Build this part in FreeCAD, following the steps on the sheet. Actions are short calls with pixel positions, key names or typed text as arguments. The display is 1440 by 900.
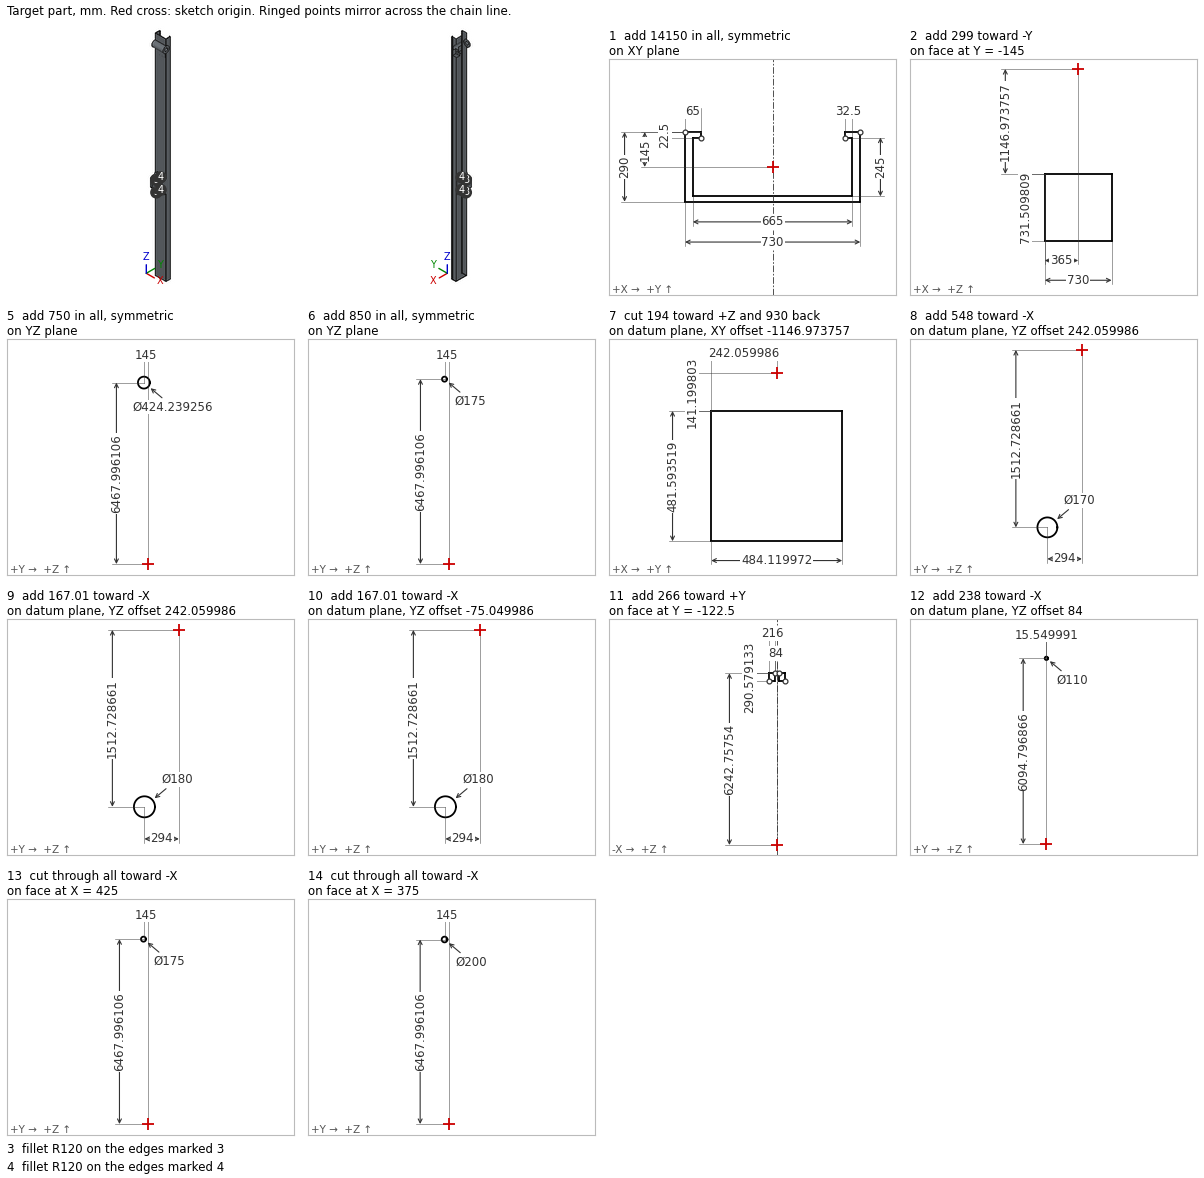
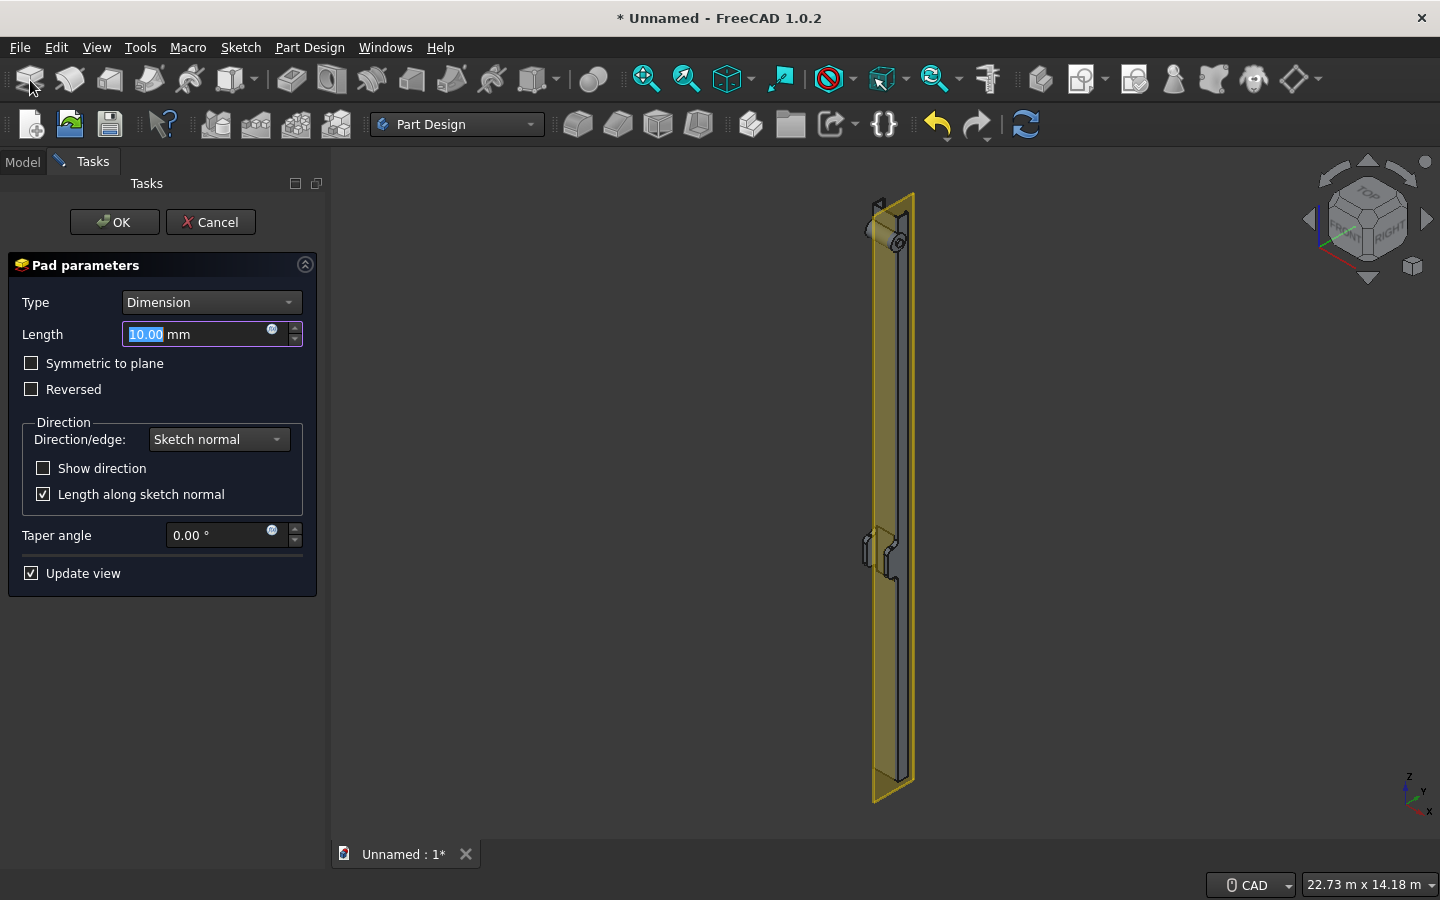
text(548)
key(Tab)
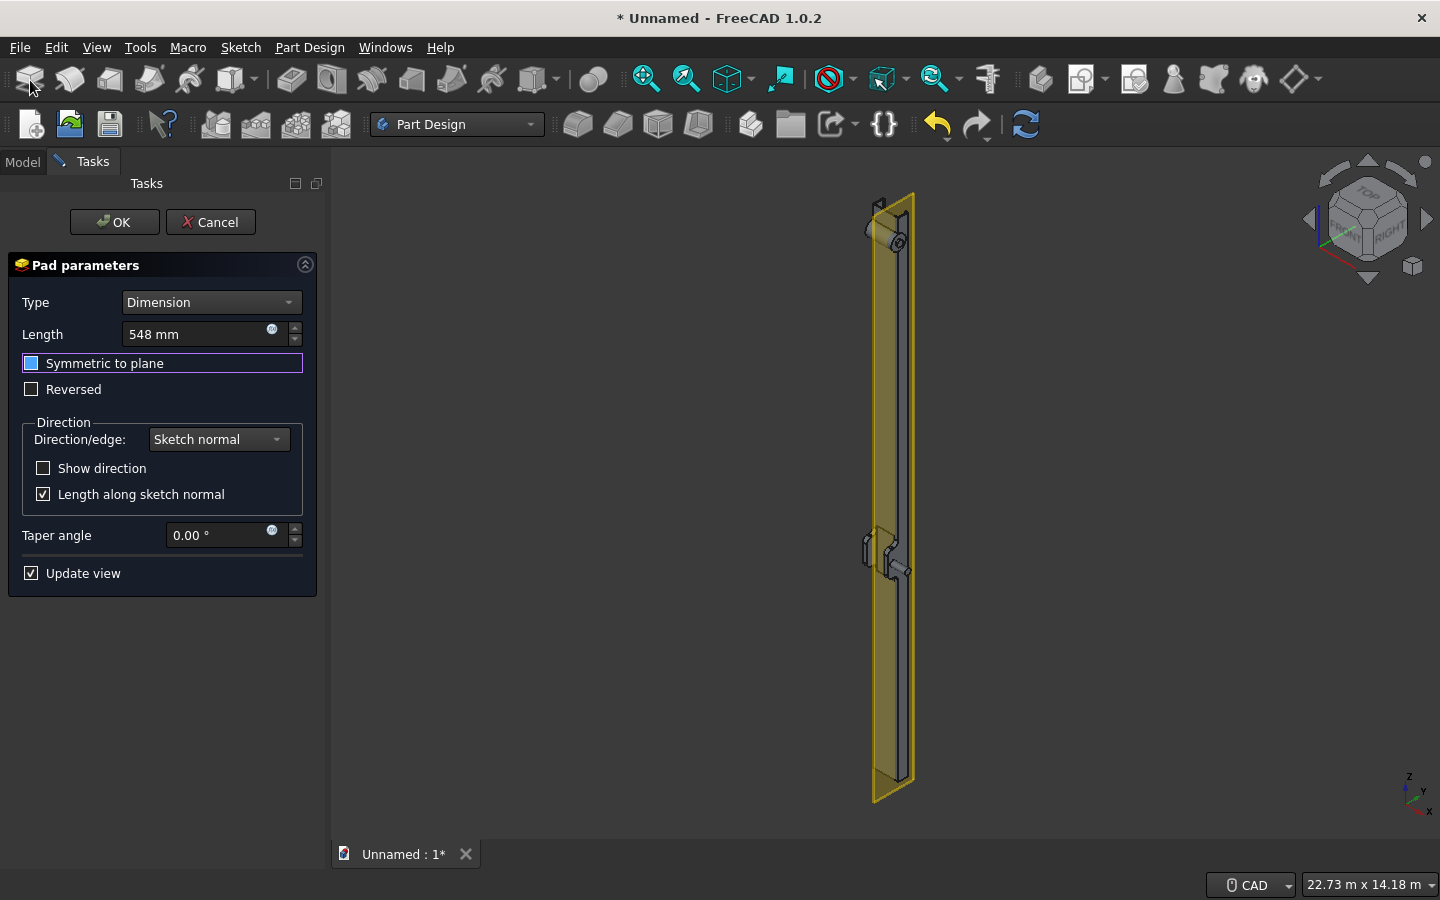
click(30, 389)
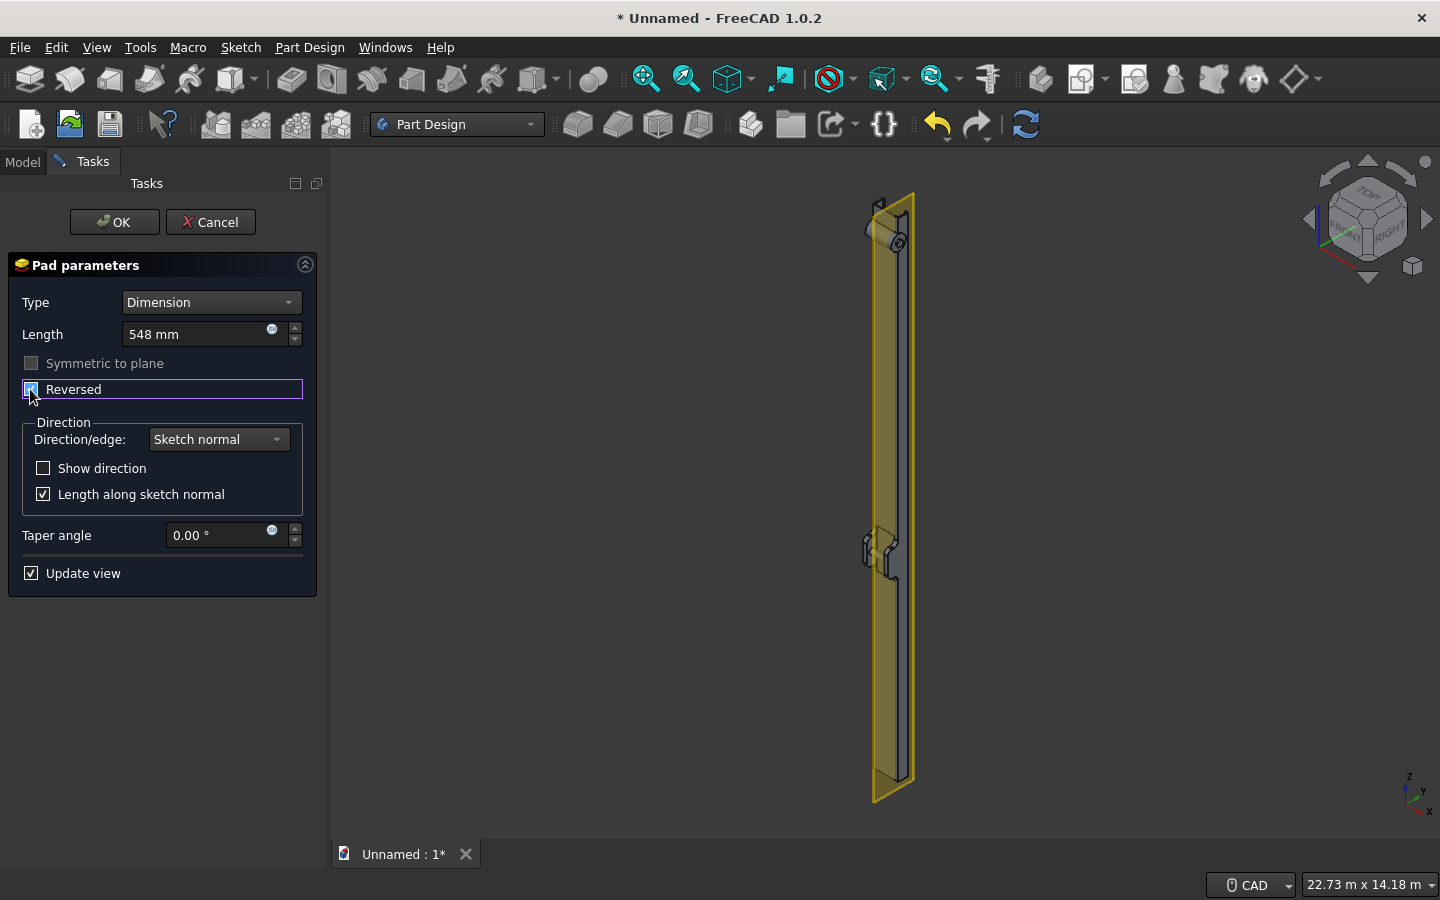
click(115, 222)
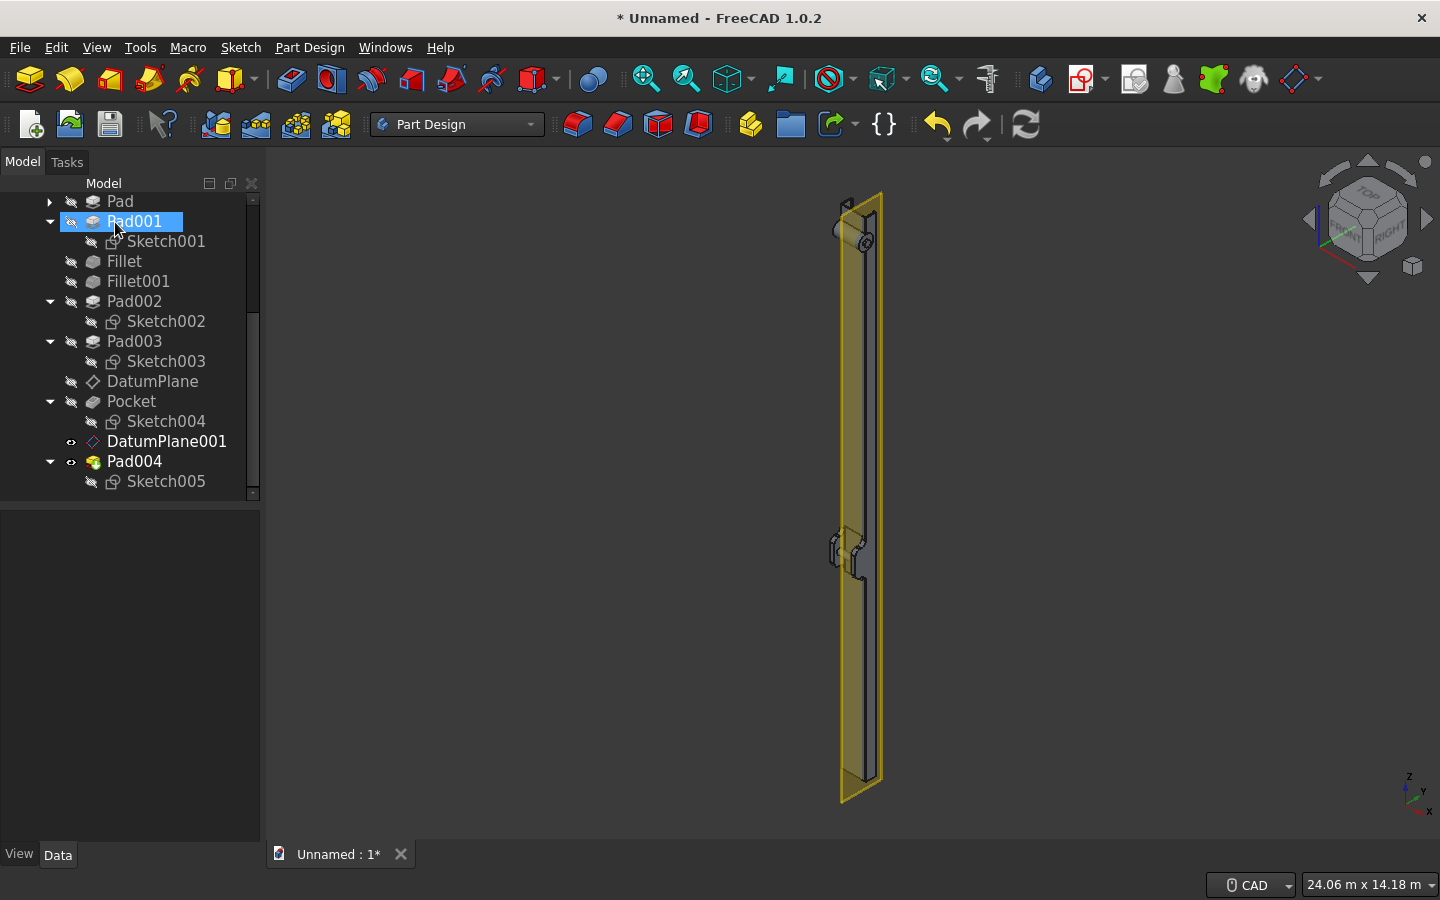
click(116, 442)
key(space)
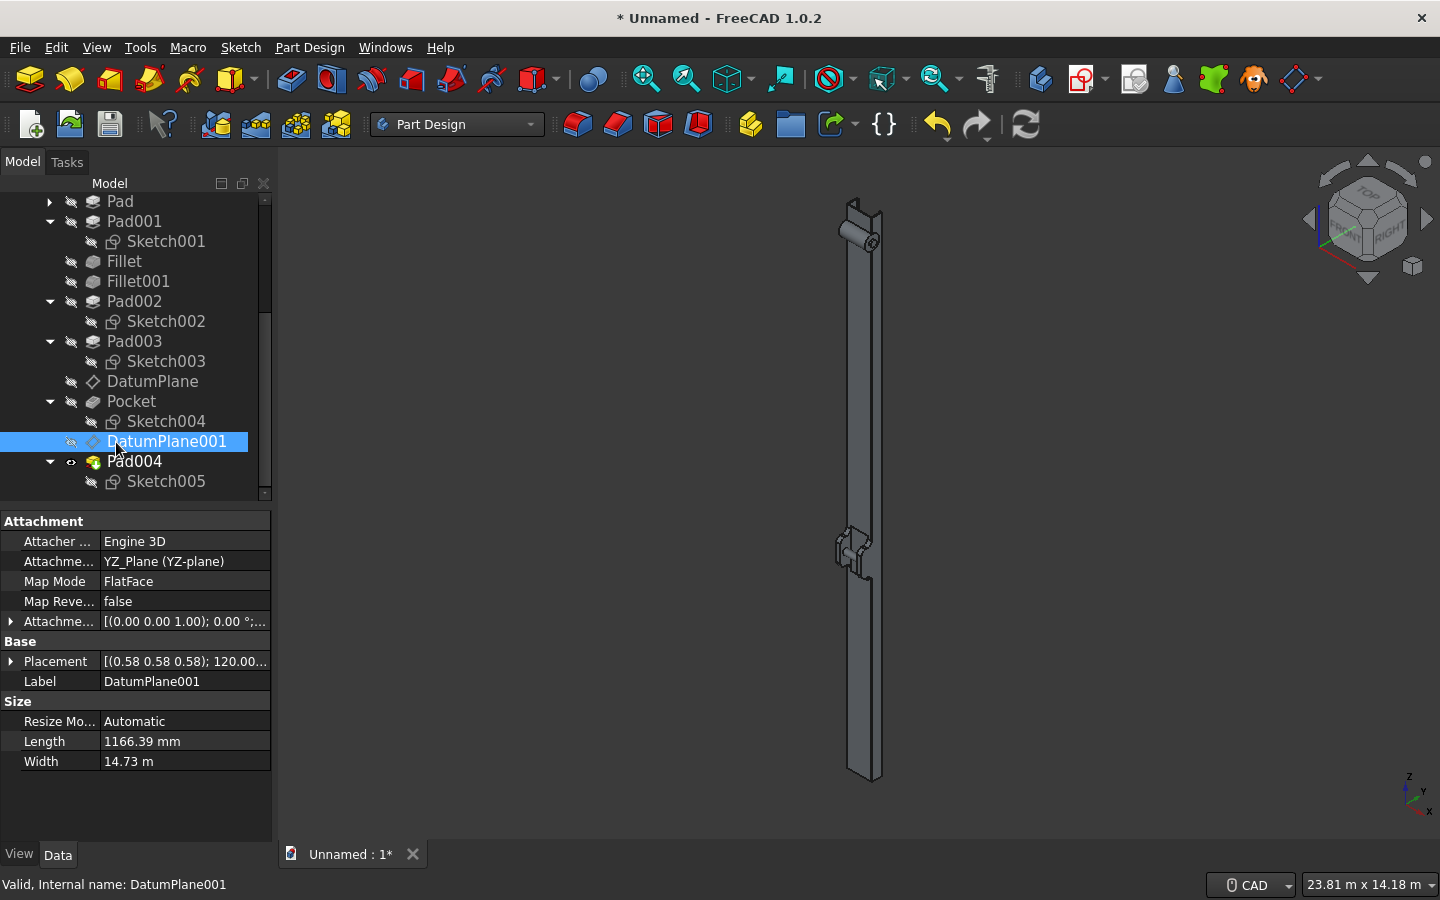
scroll(140, 337, down, 3)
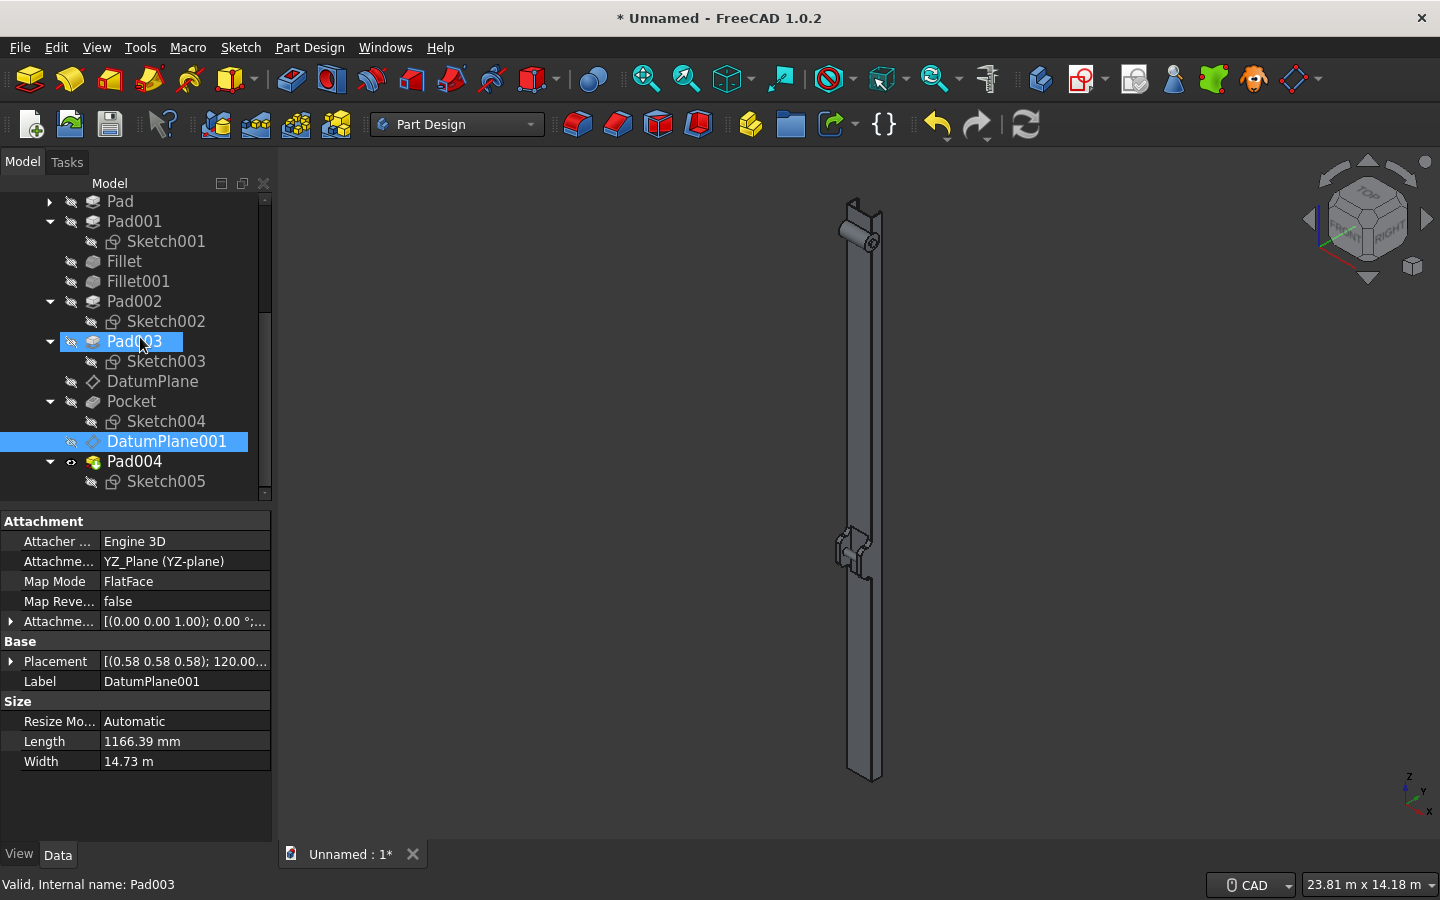
scroll(140, 337, up, 15)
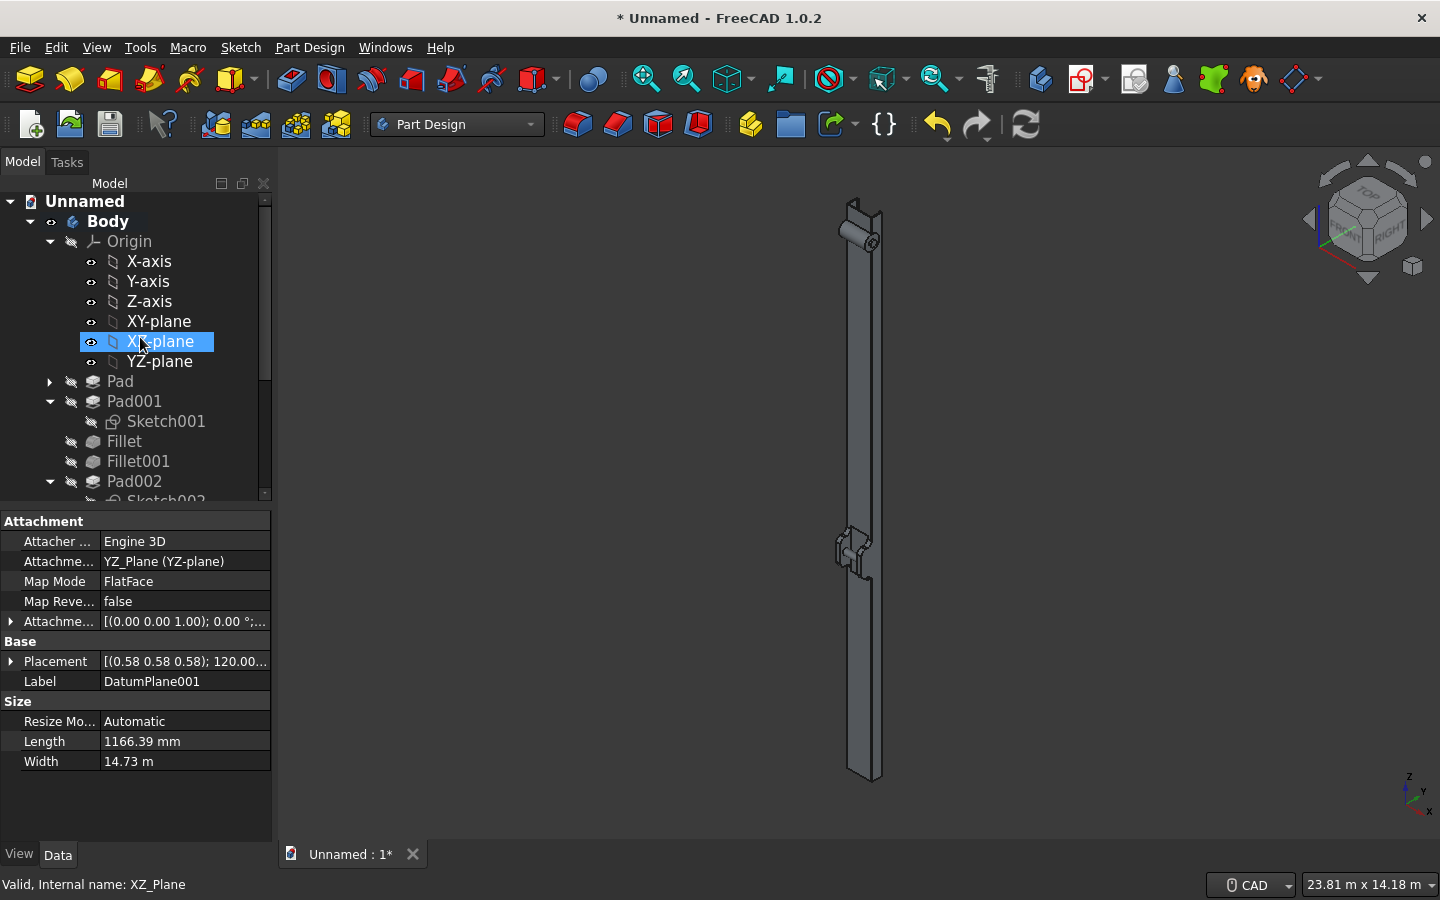
click(136, 362)